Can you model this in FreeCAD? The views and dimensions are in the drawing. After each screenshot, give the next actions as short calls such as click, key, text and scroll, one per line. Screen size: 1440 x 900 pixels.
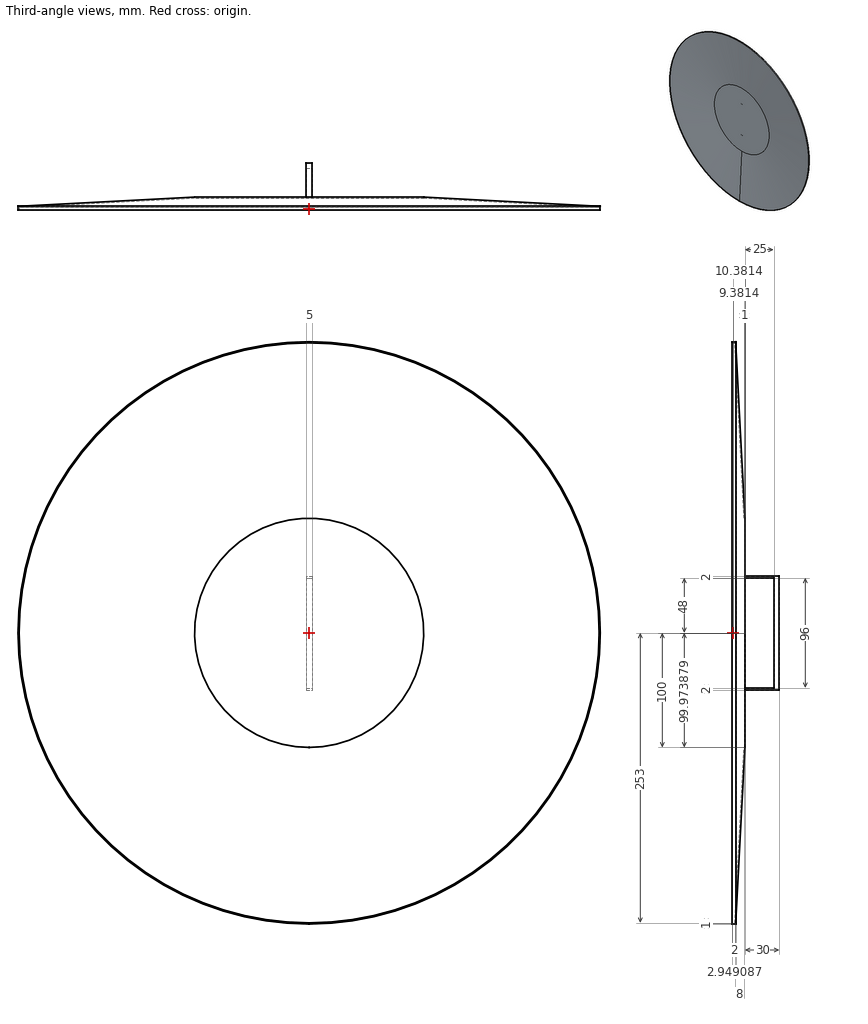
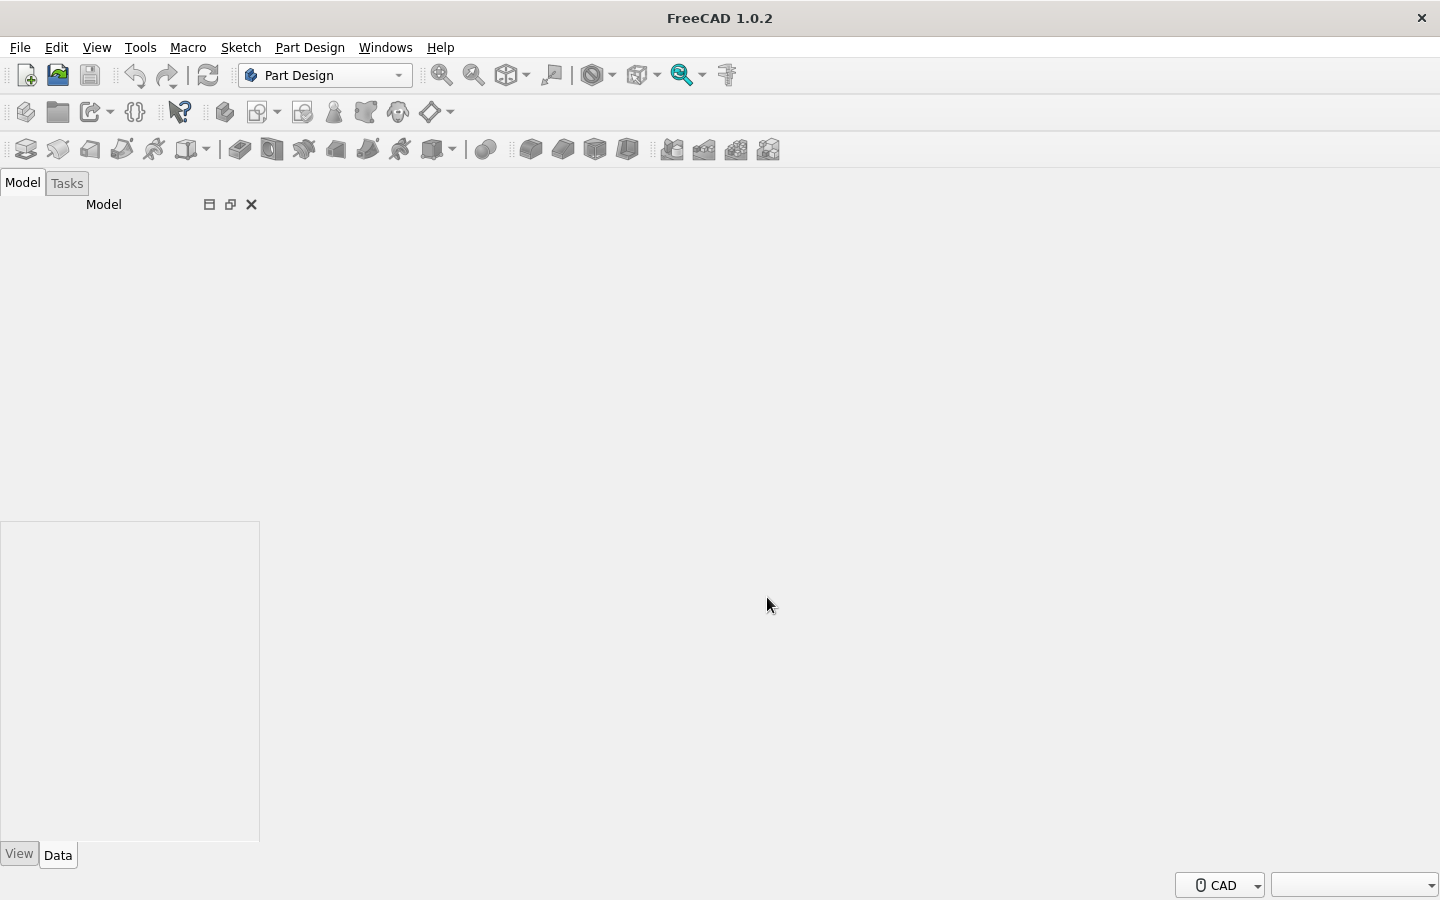
click(26, 76)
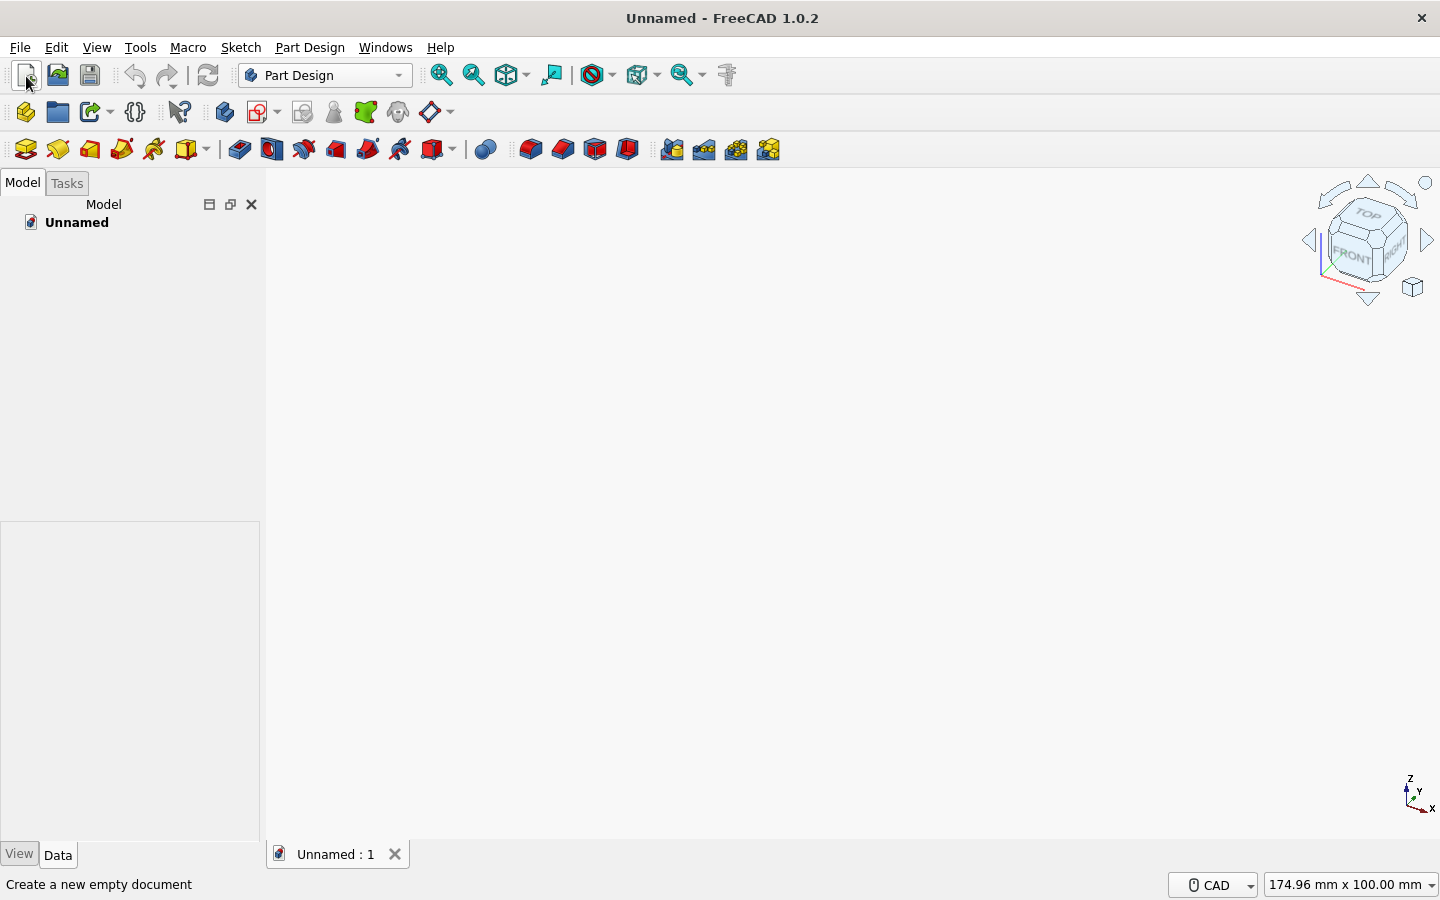
click(258, 112)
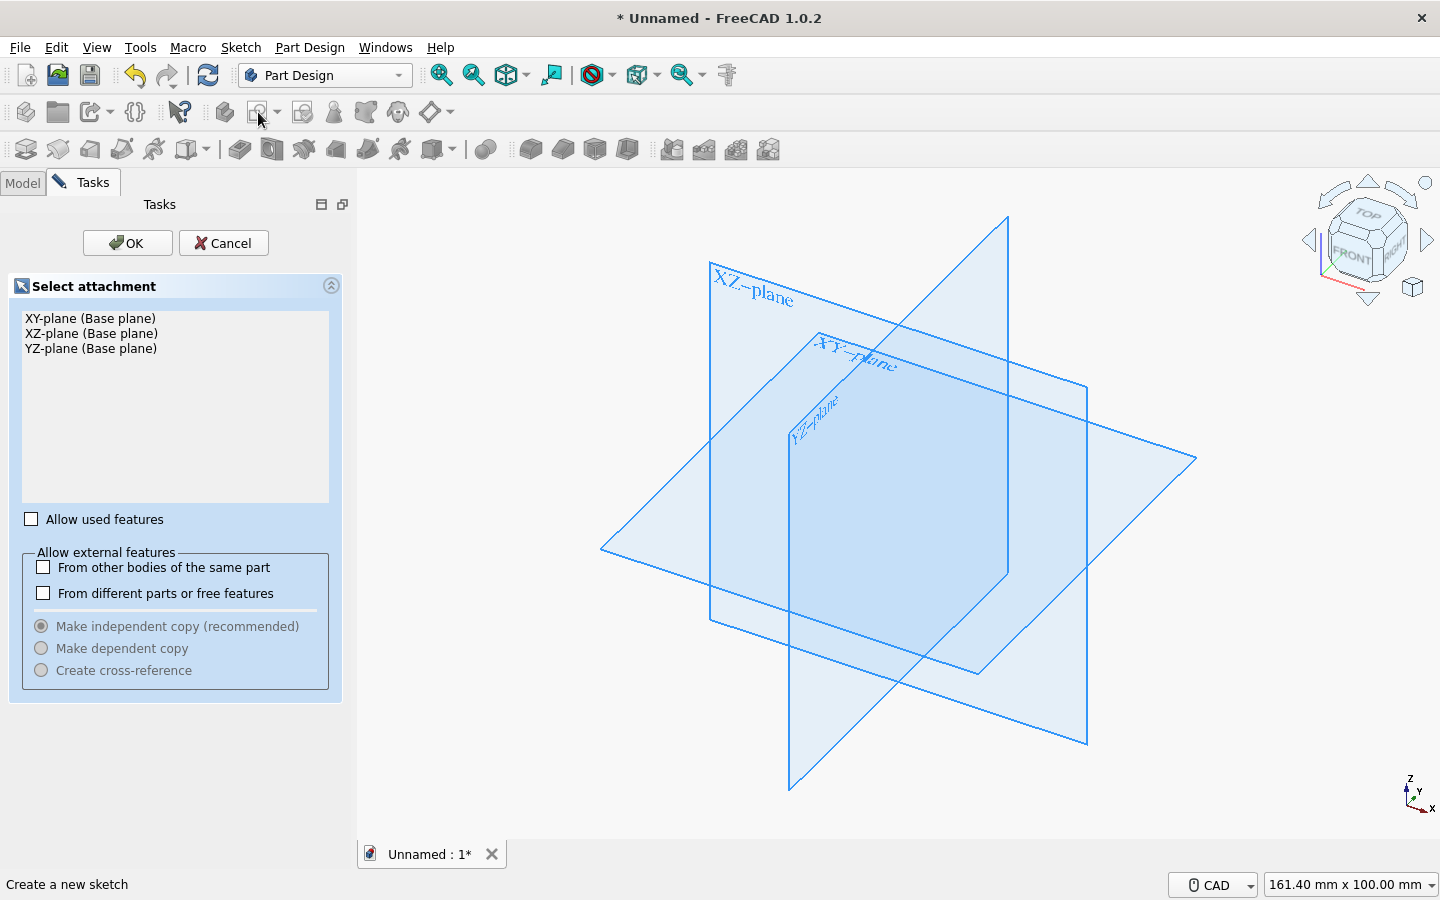
click(82, 348)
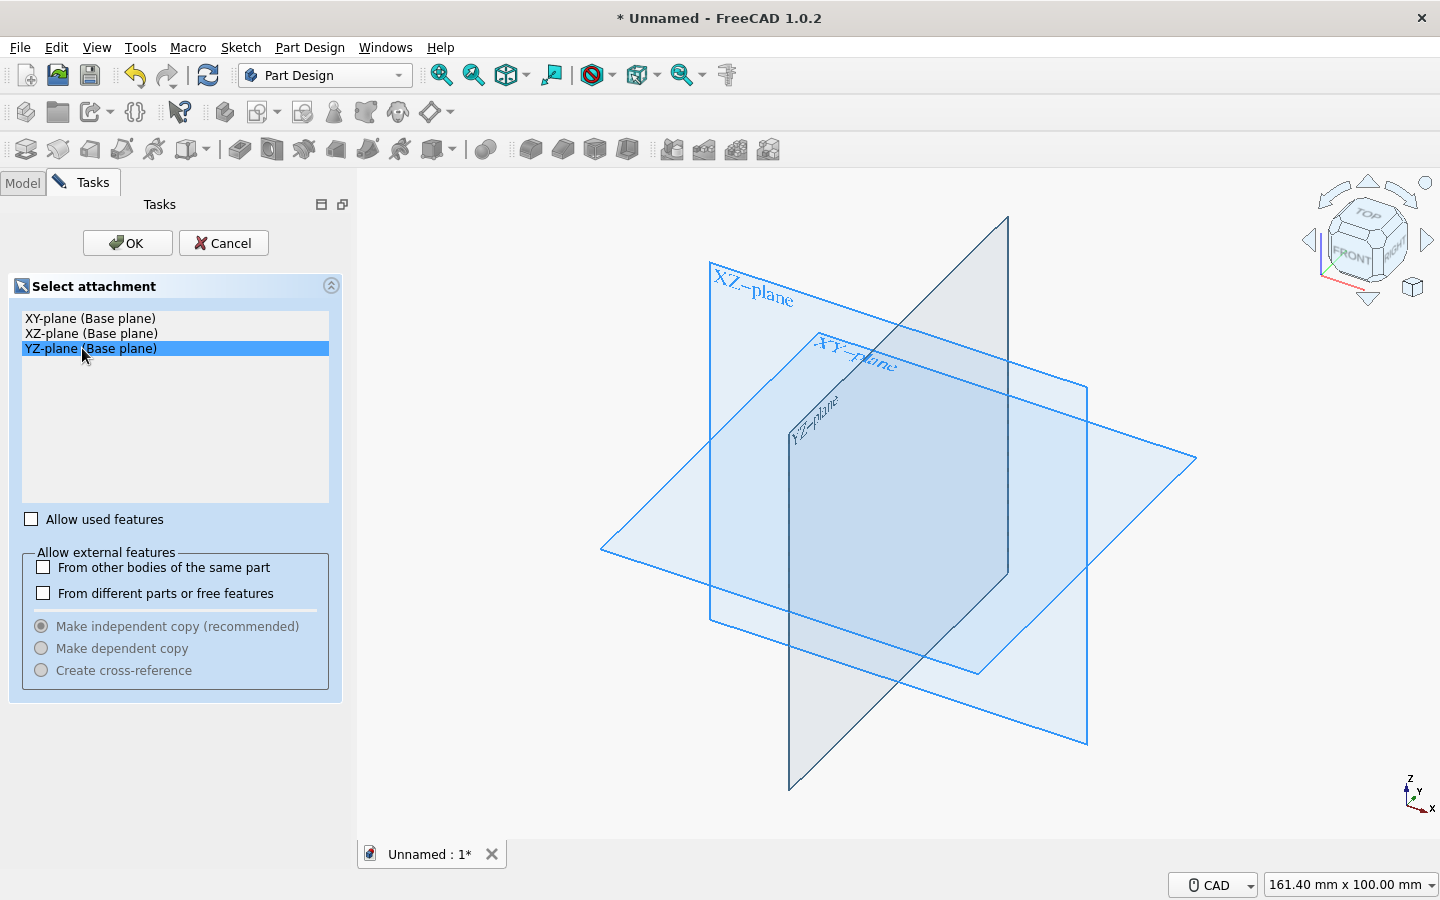
click(128, 243)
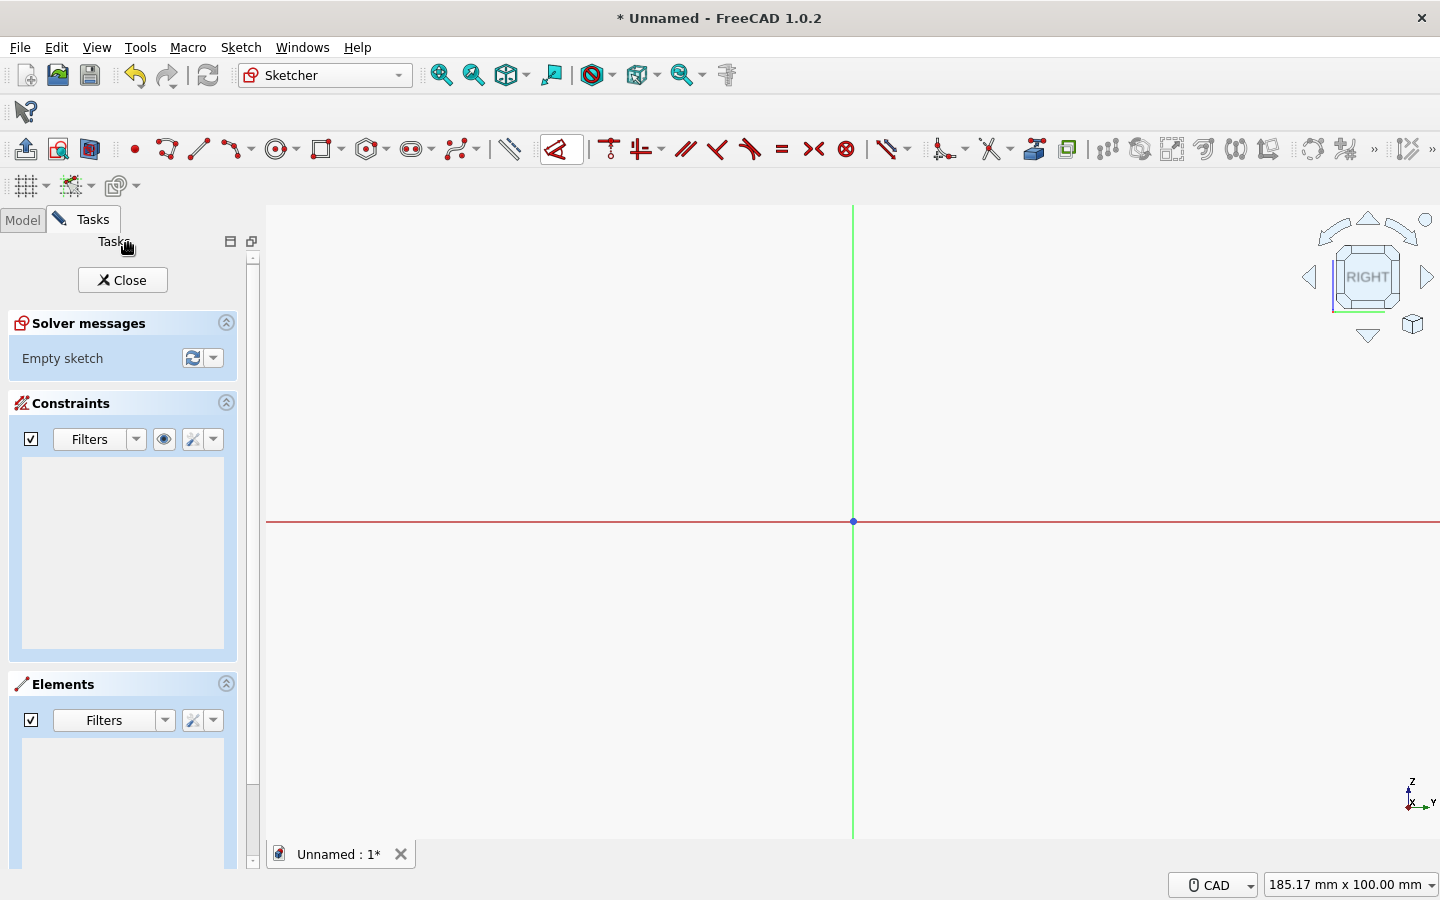
scroll(752, 258, down, 7)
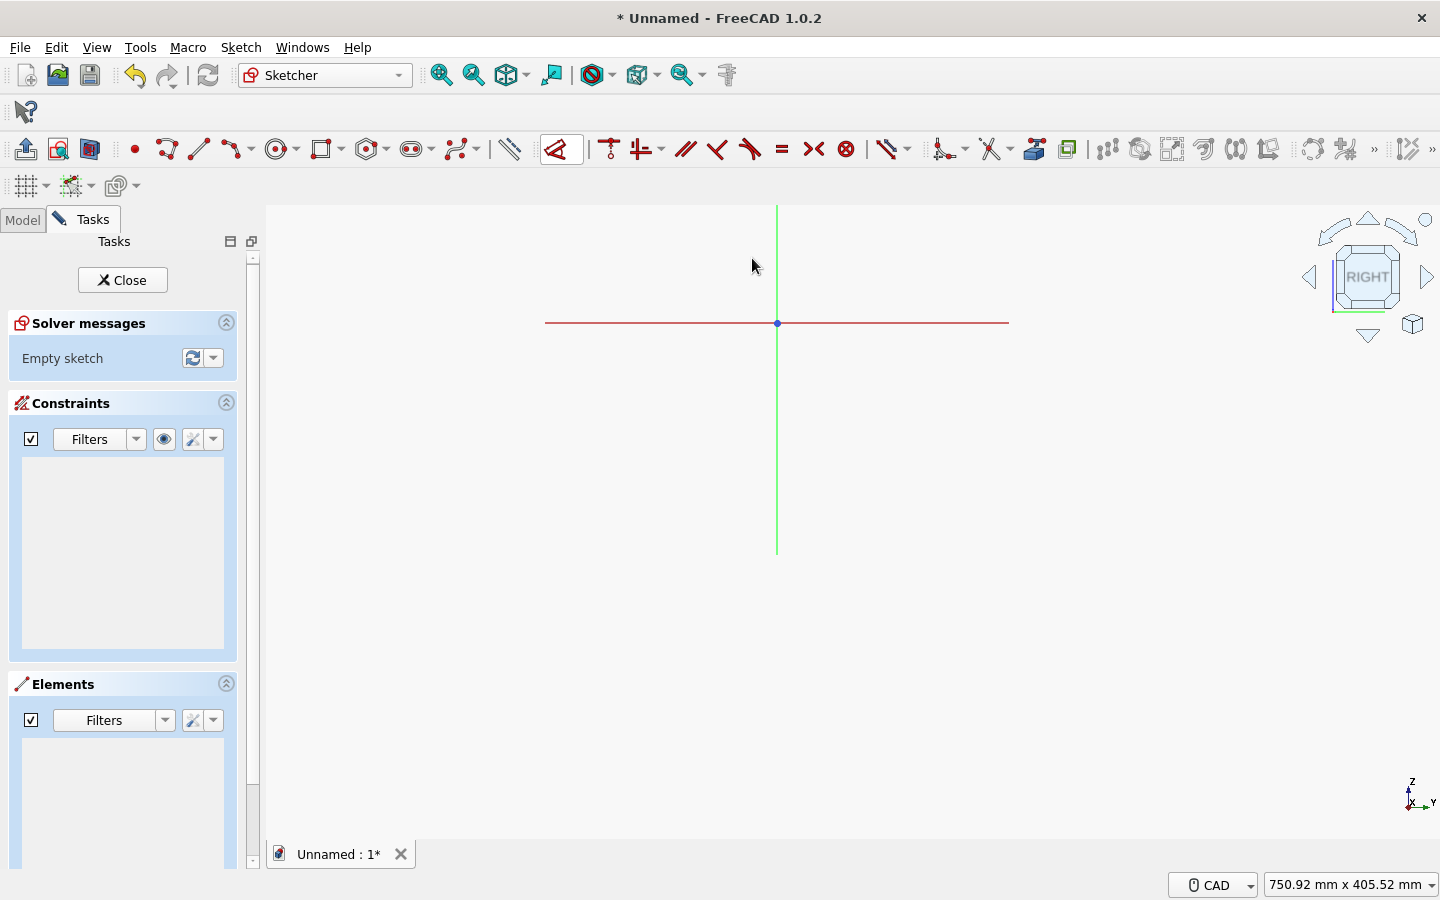
key(g)
key(m)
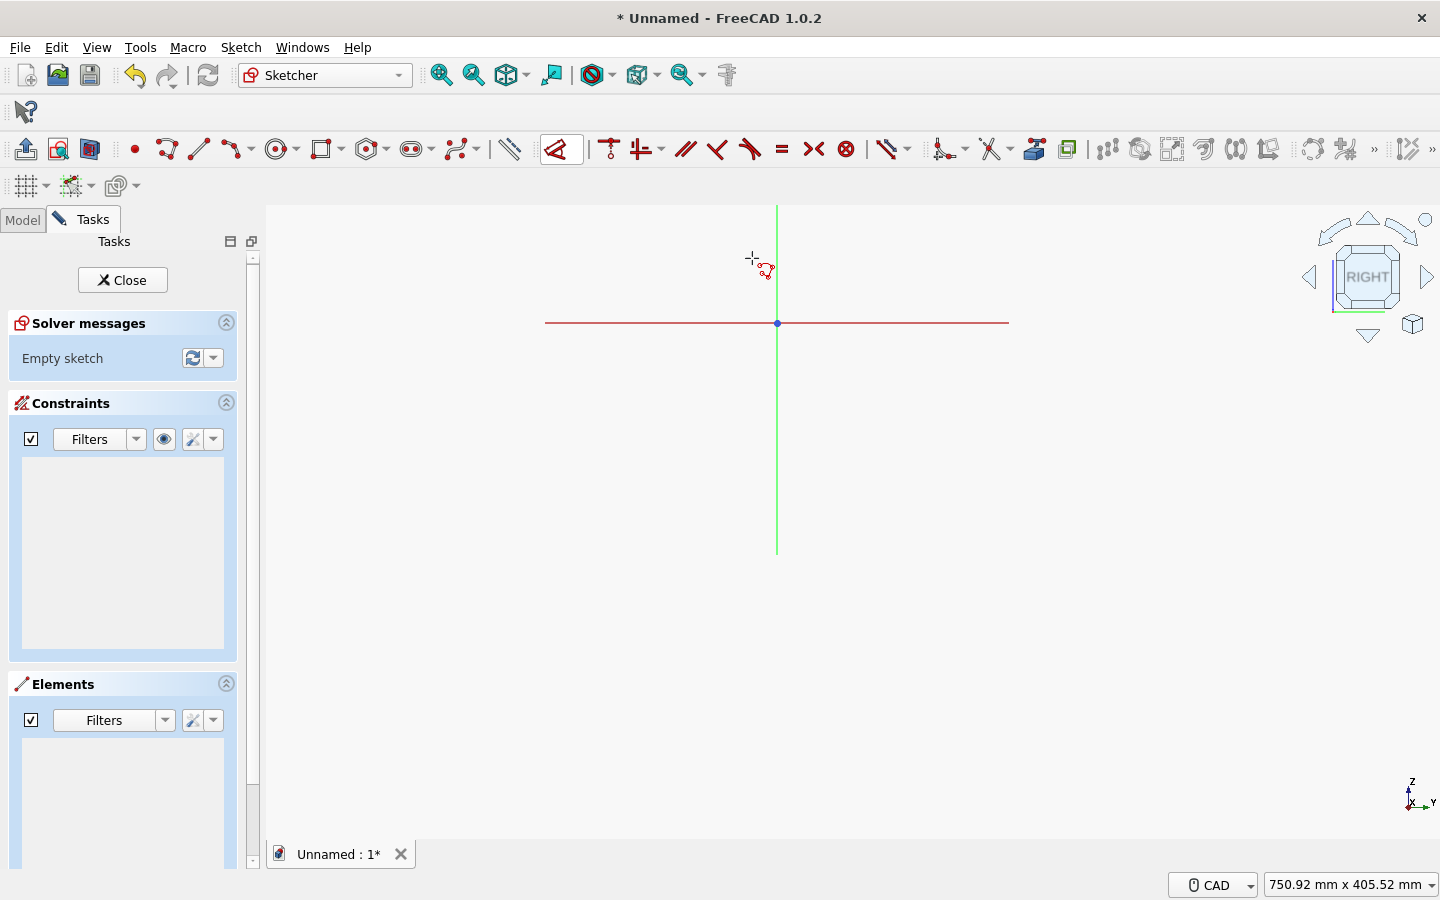
click(792, 323)
click(792, 479)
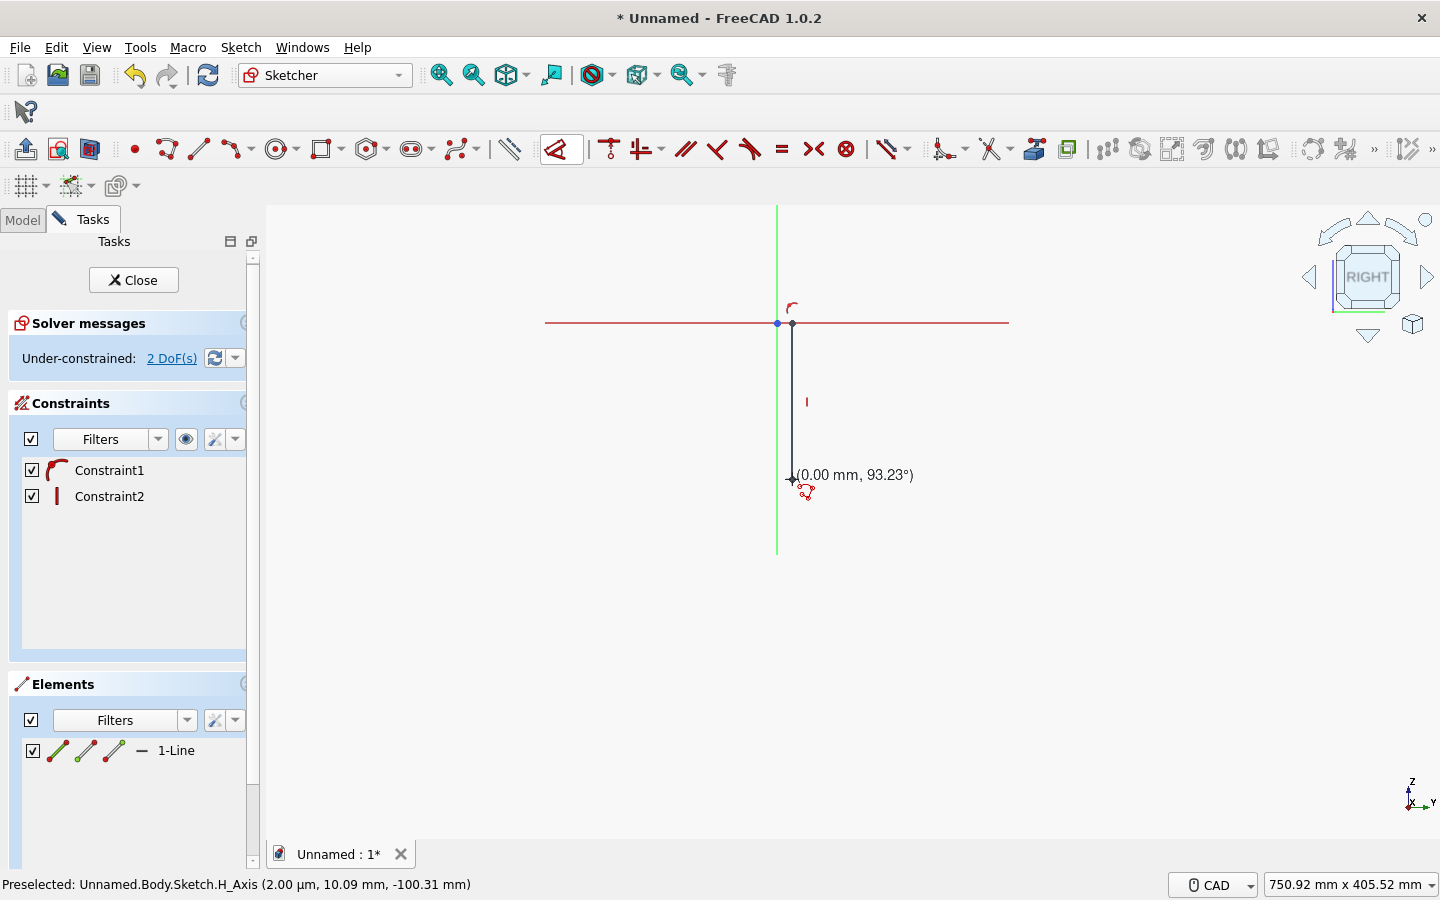
scroll(779, 719, up, 10)